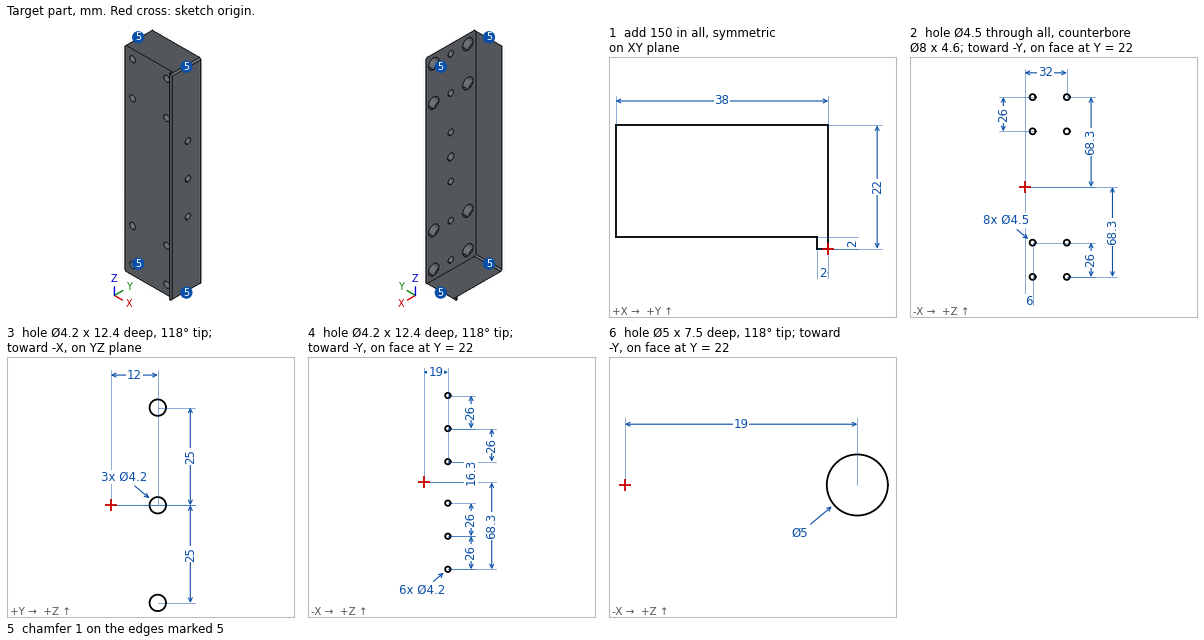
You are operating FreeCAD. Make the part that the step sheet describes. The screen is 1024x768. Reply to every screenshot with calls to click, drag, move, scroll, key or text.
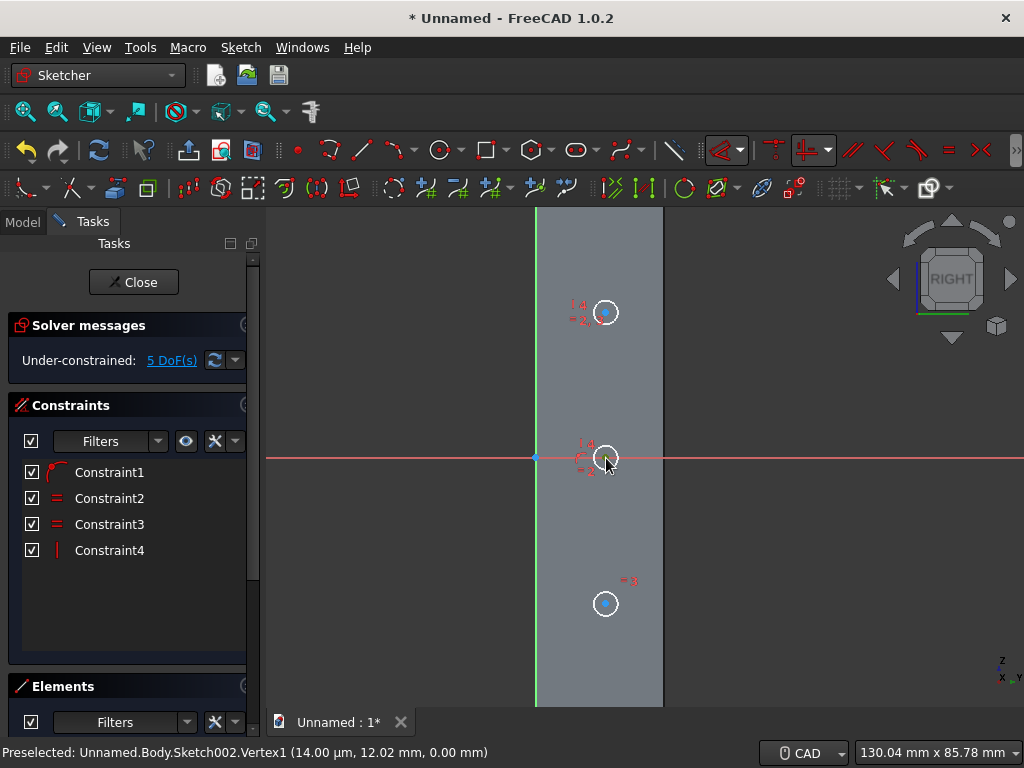
click(606, 604)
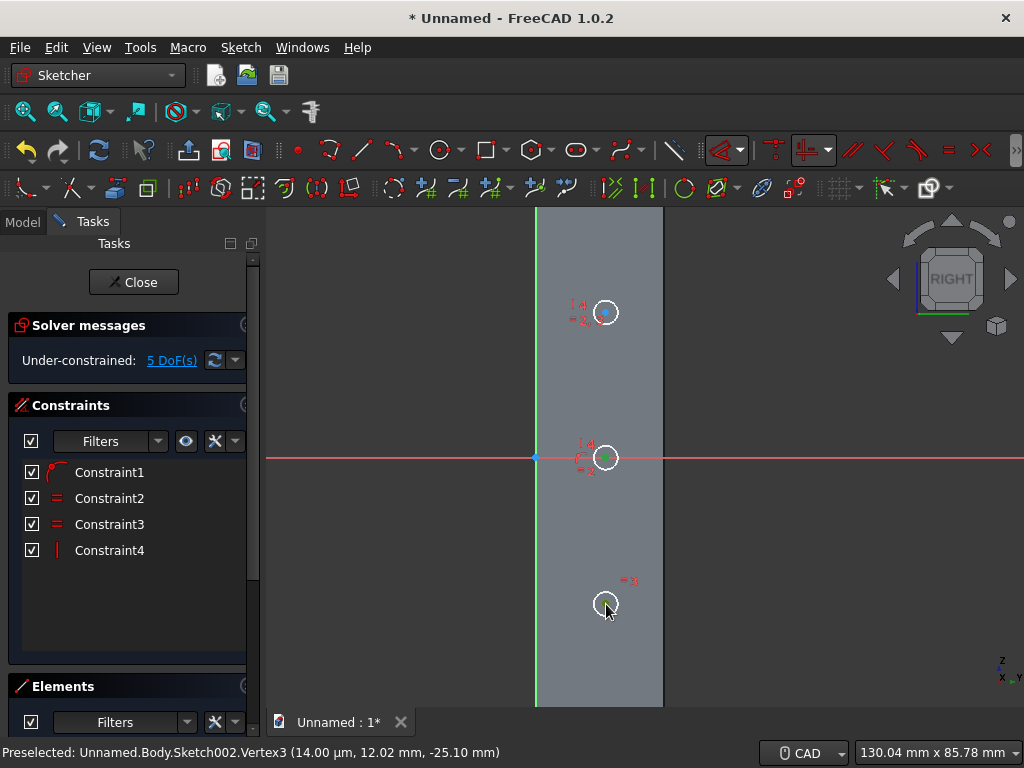
key(v)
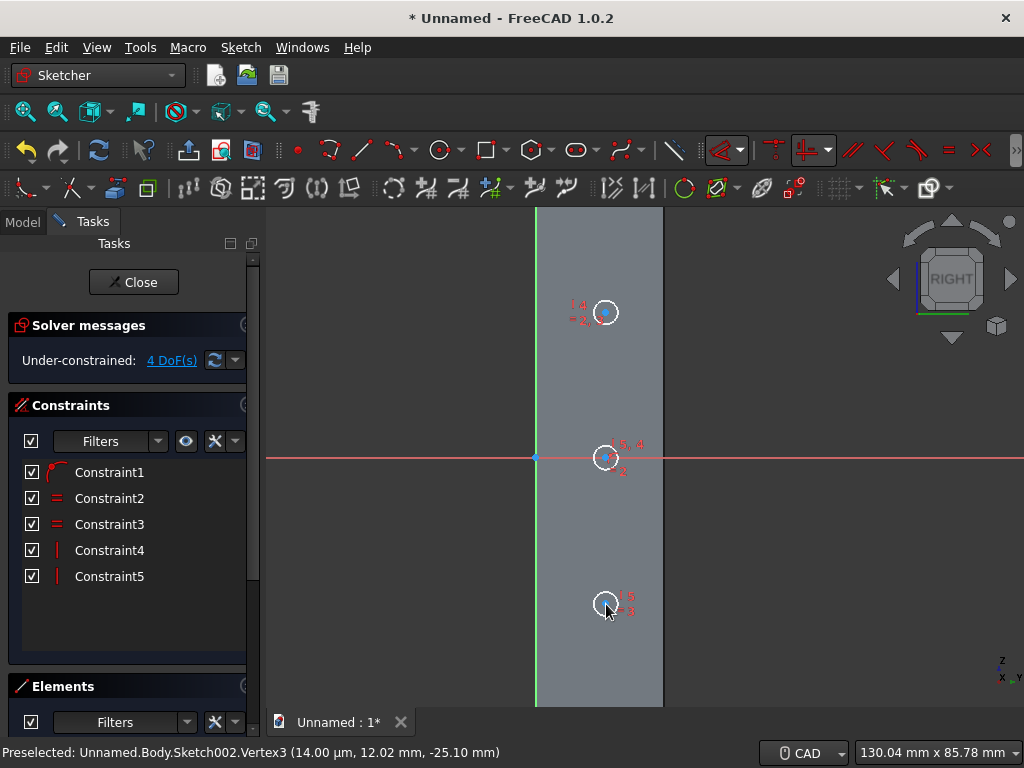
scroll(606, 446, up, 3)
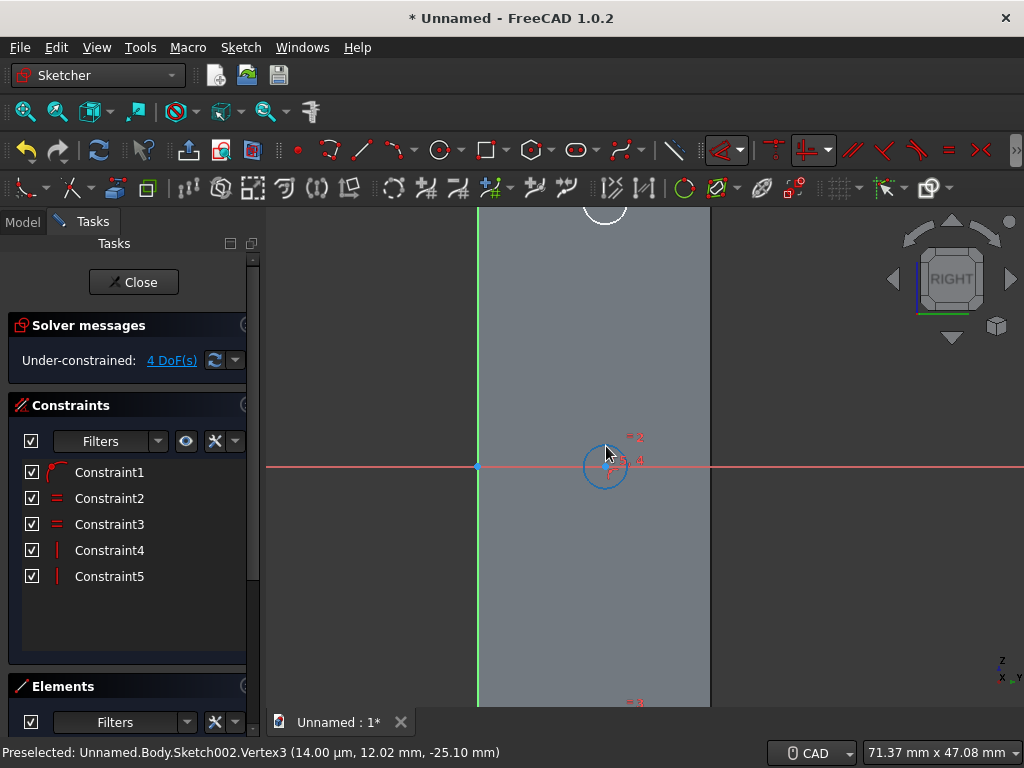
click(606, 445)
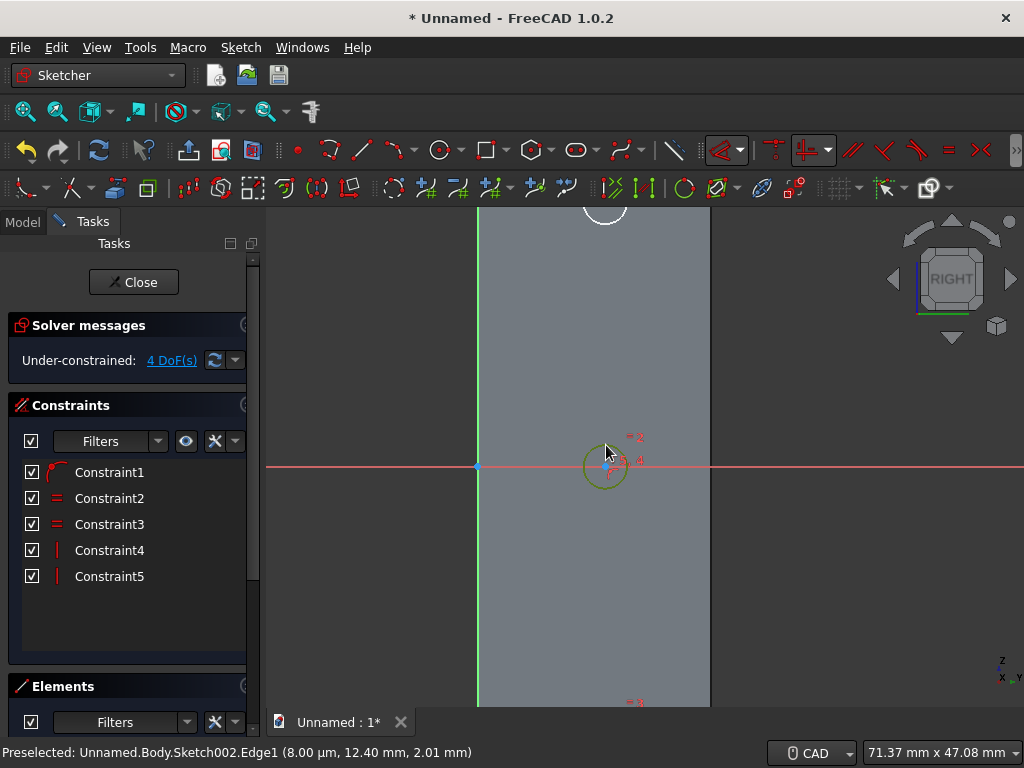
key(k)
key(o)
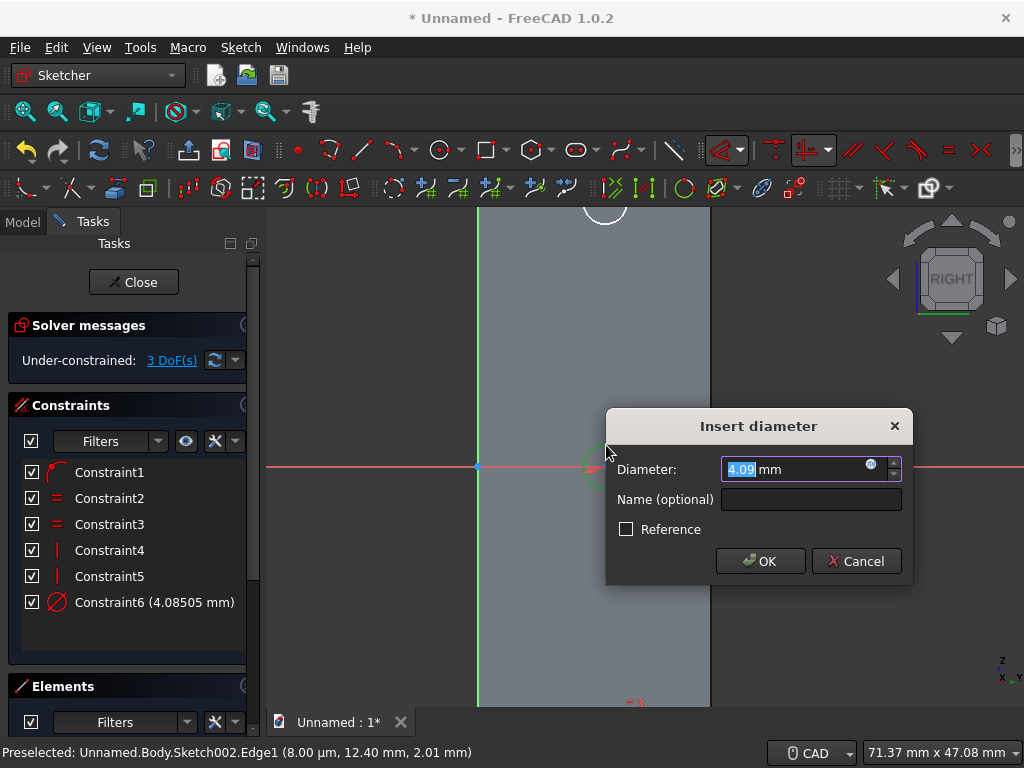
text(4.2)
key(Return)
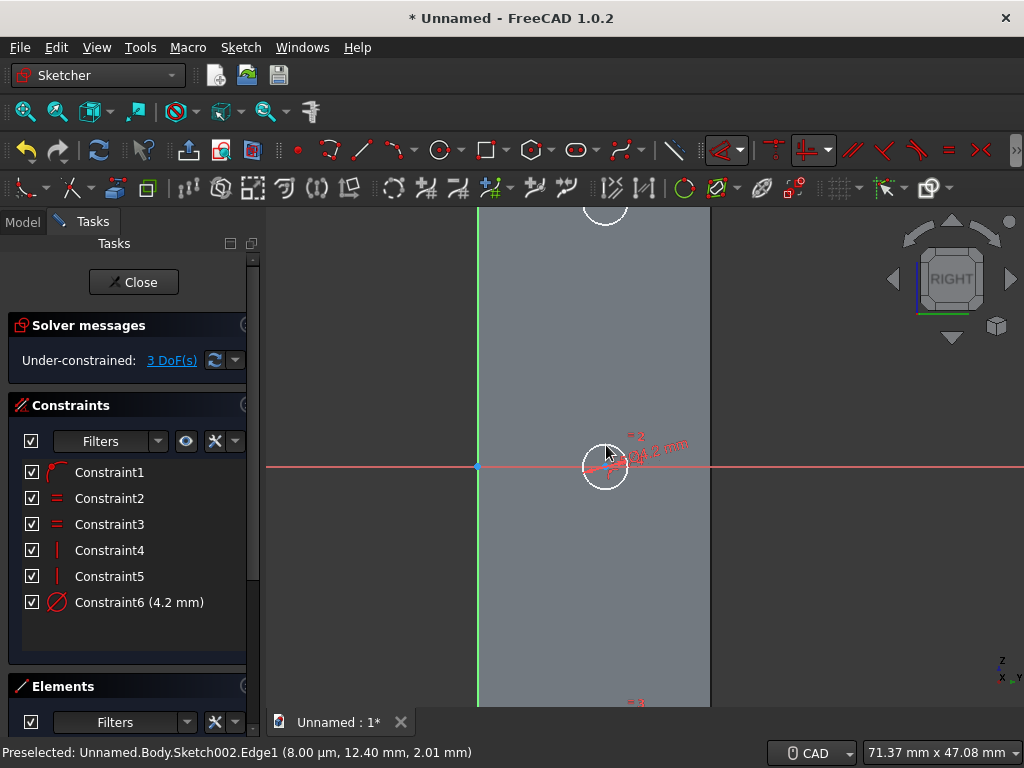
click(605, 467)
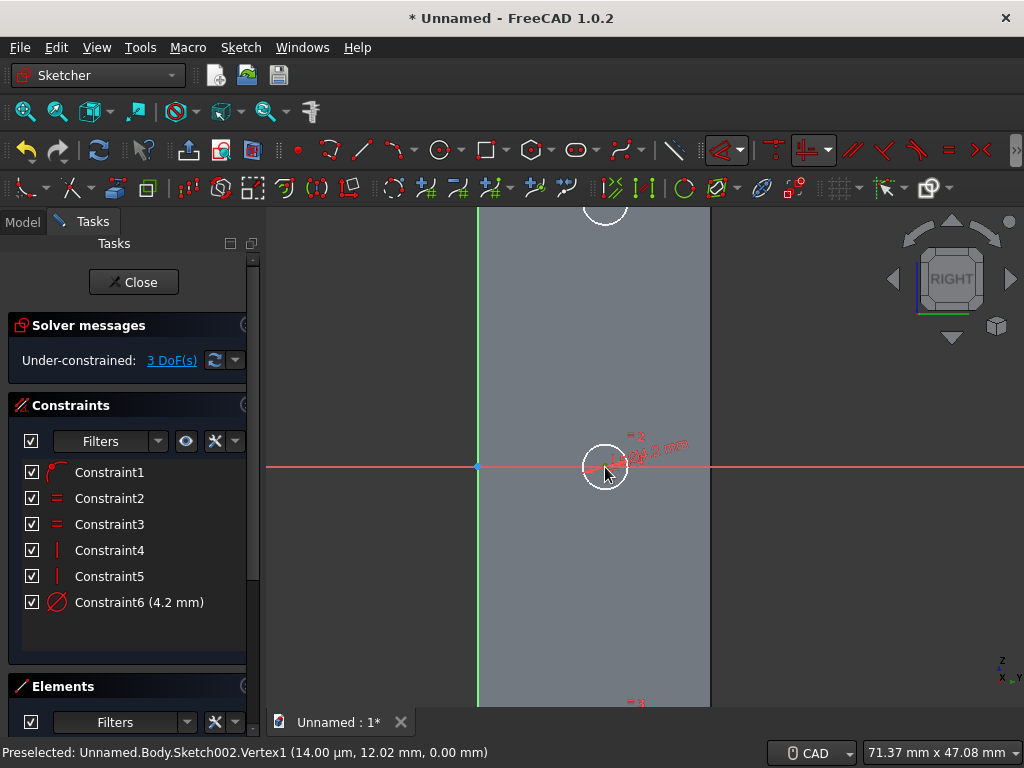
key(l)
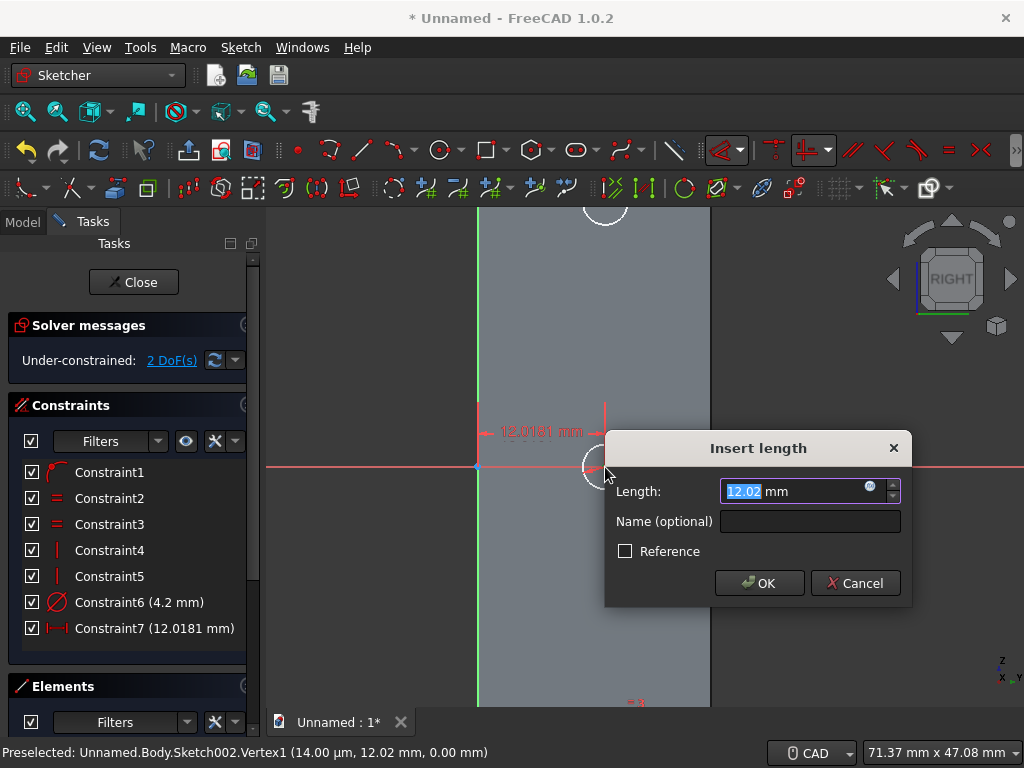
text(12)
key(Return)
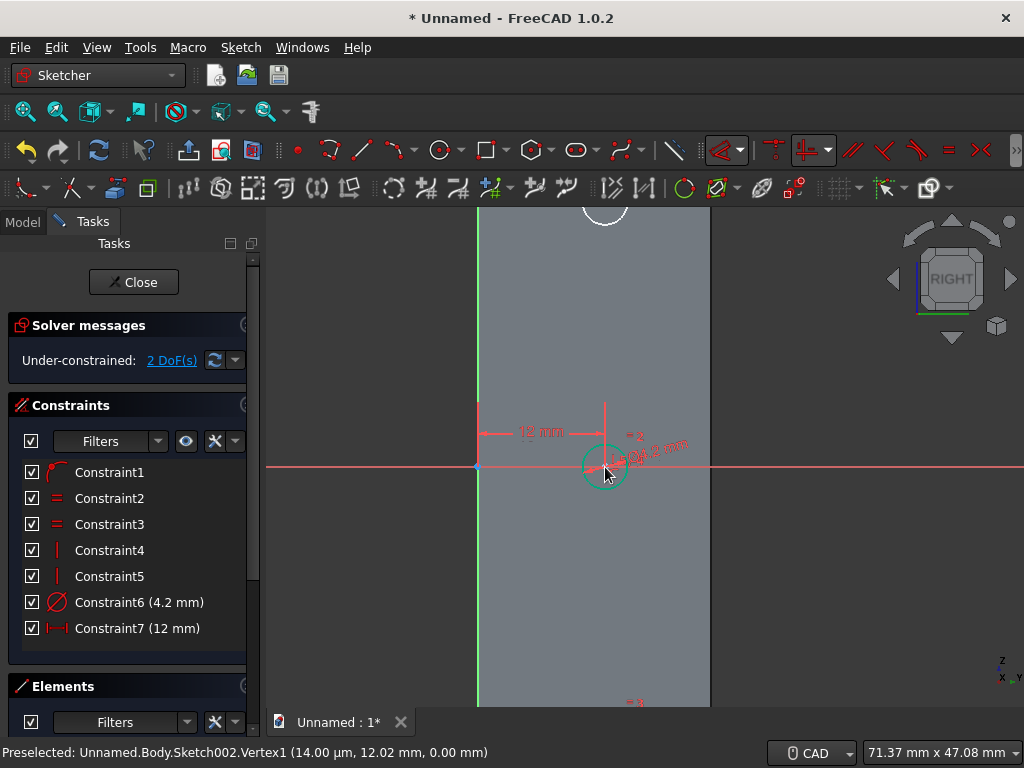
scroll(606, 445, down, 3)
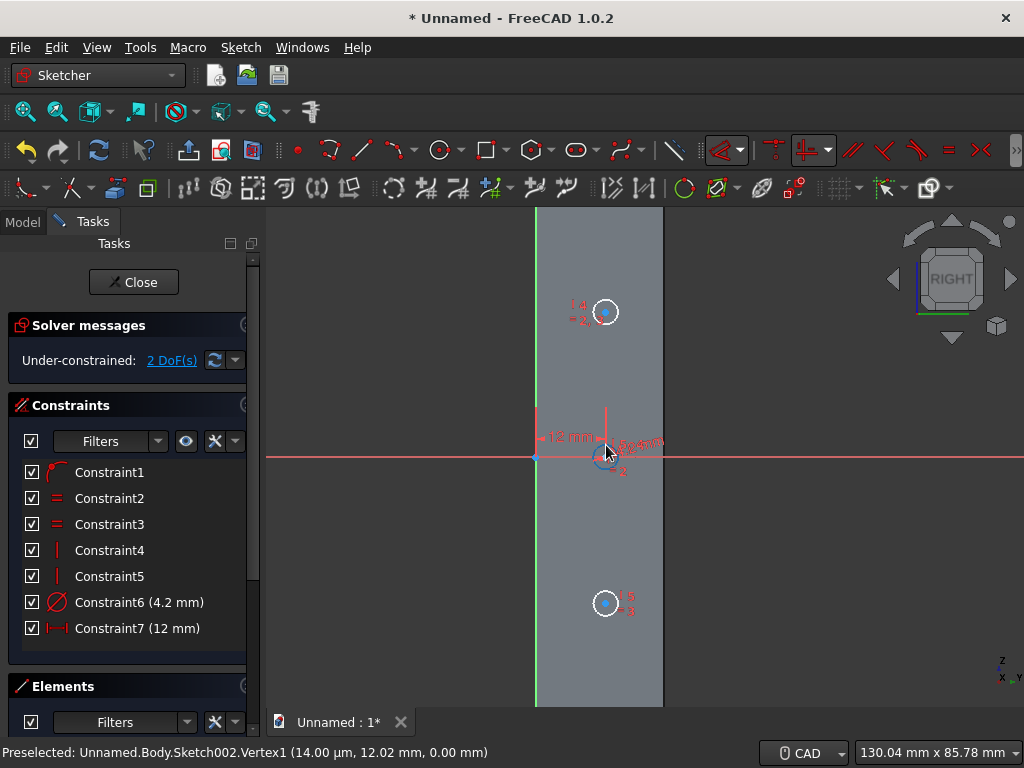
click(606, 312)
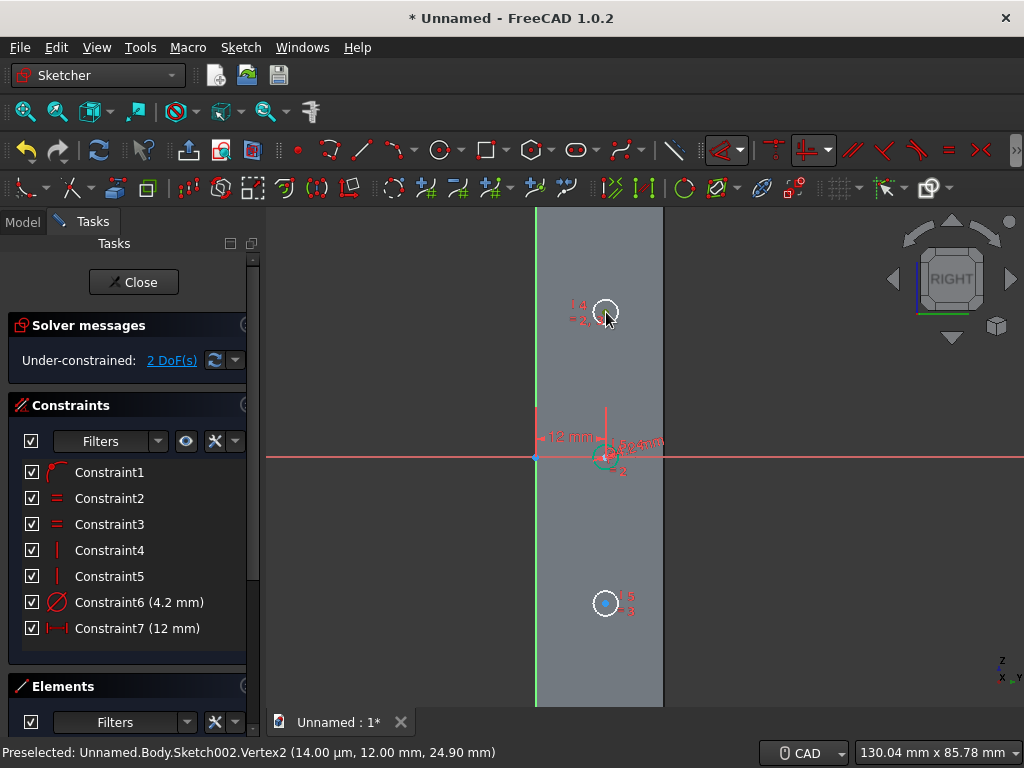
key(i)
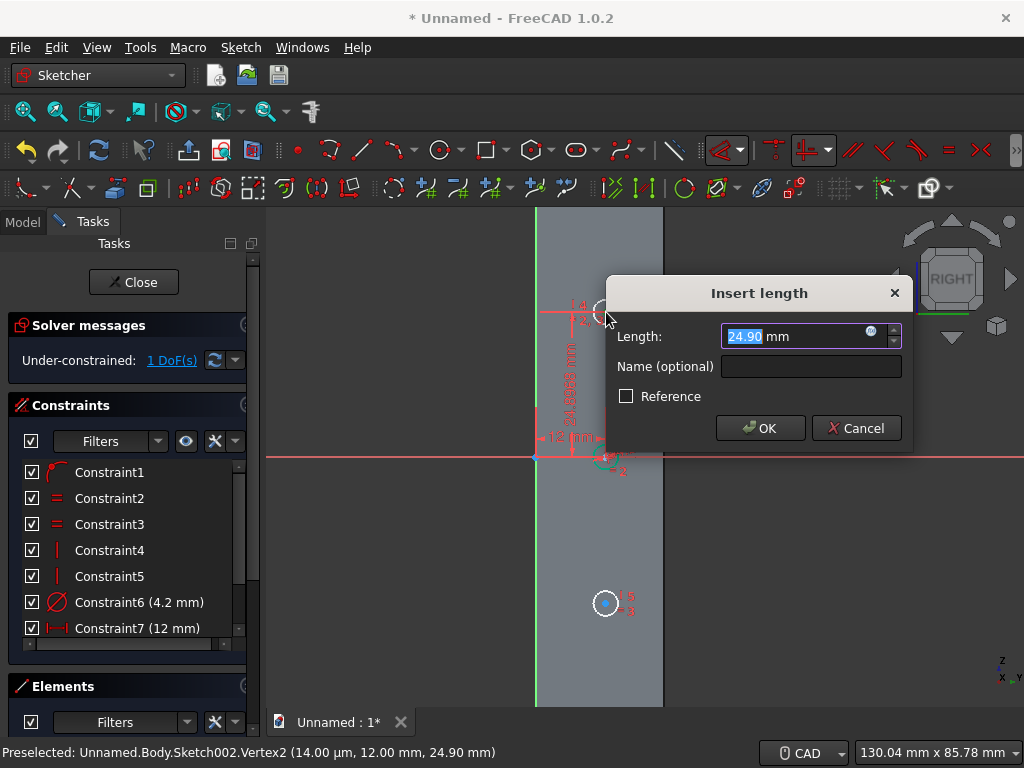
text(25)
key(Return)